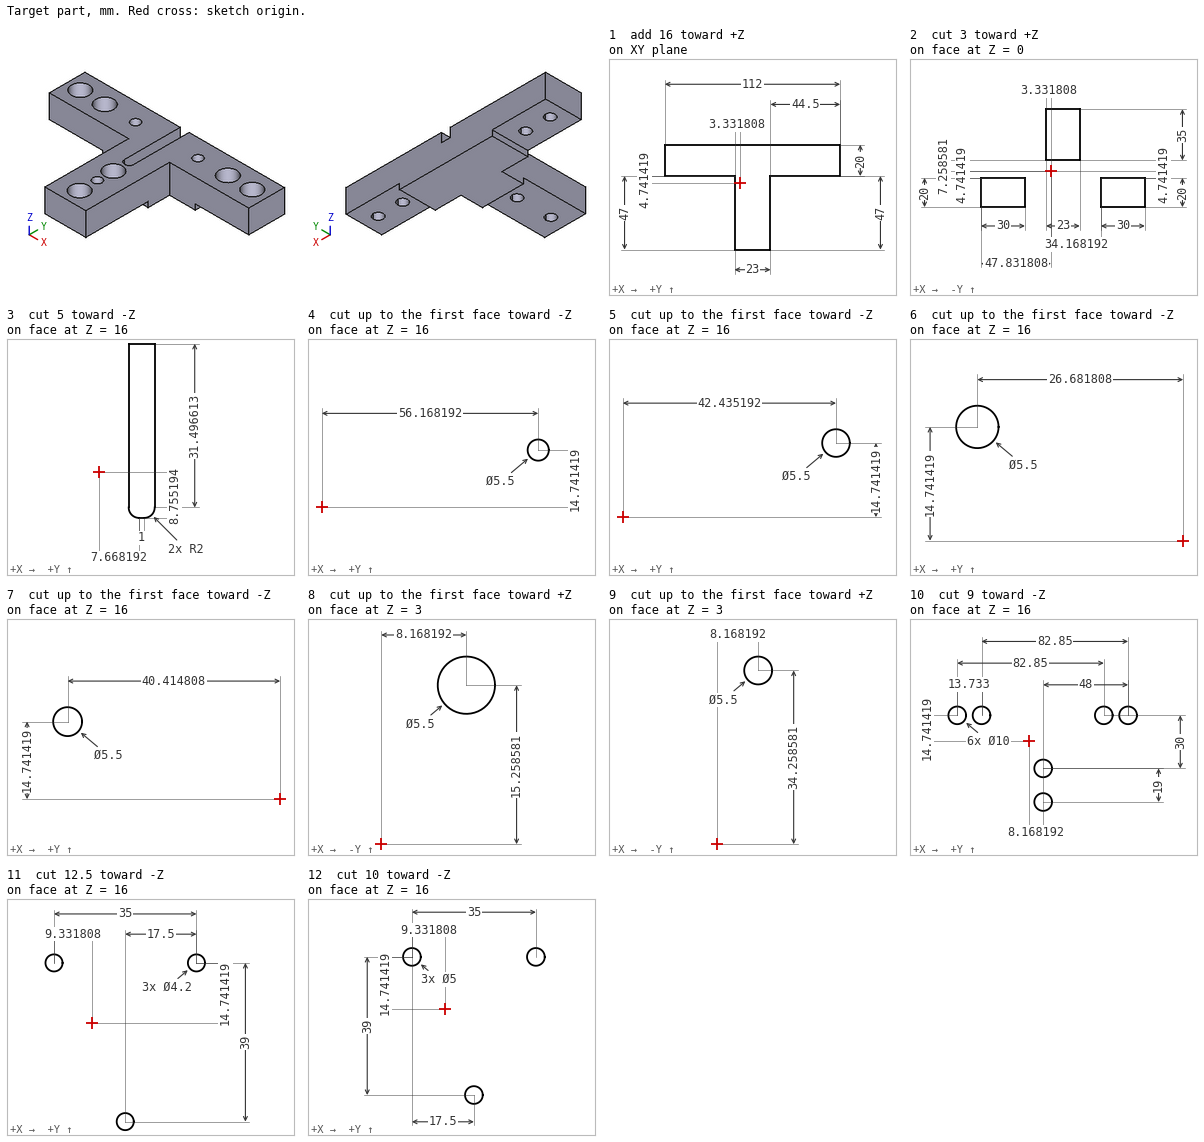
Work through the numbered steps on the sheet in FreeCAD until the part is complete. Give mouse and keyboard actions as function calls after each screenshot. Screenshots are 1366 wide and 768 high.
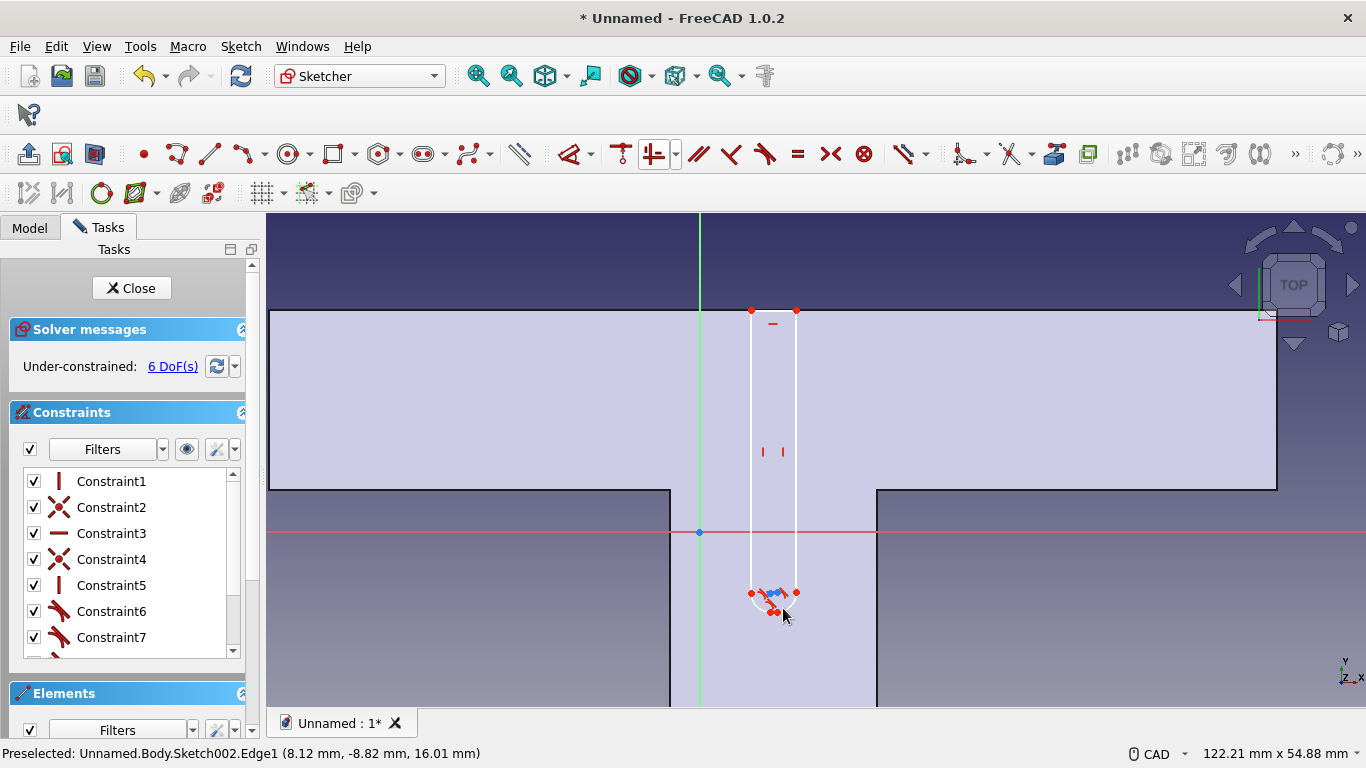
scroll(786, 610, up, 3)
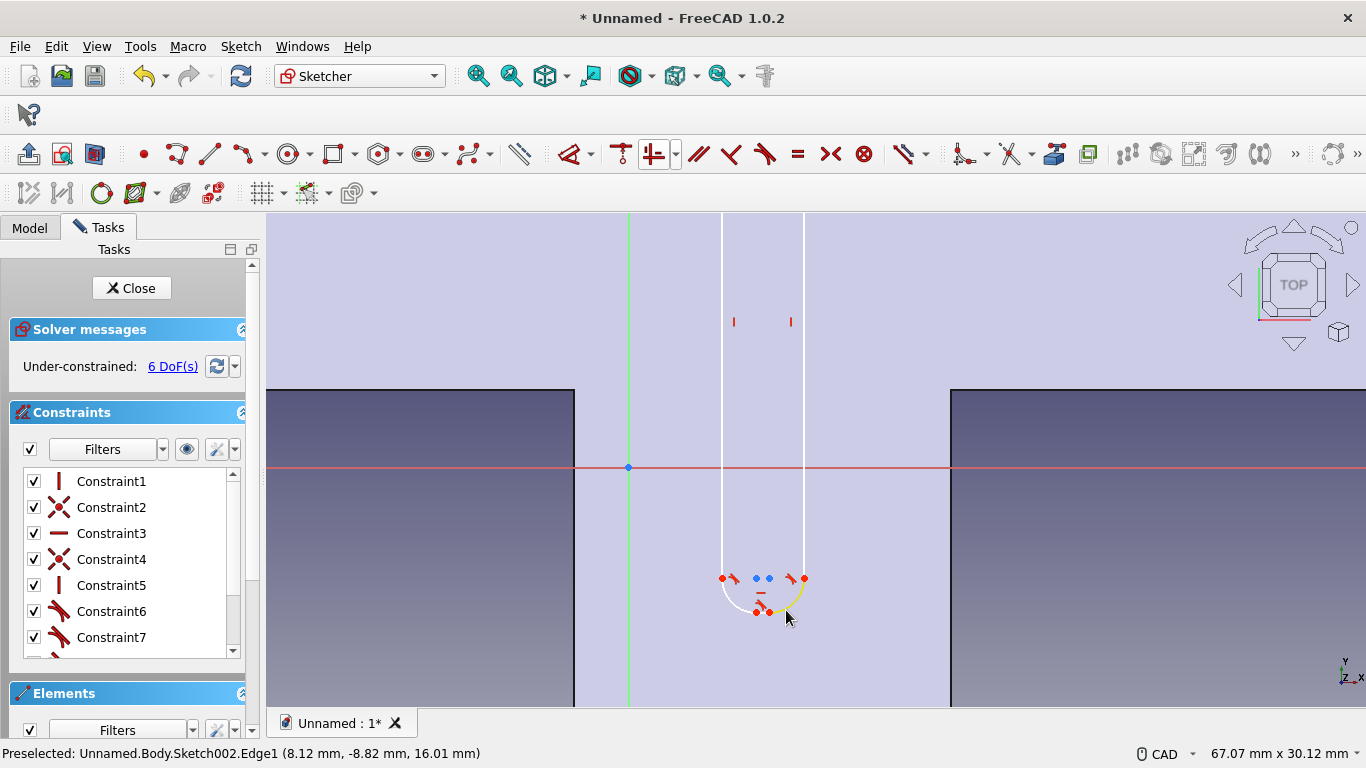
click(785, 609)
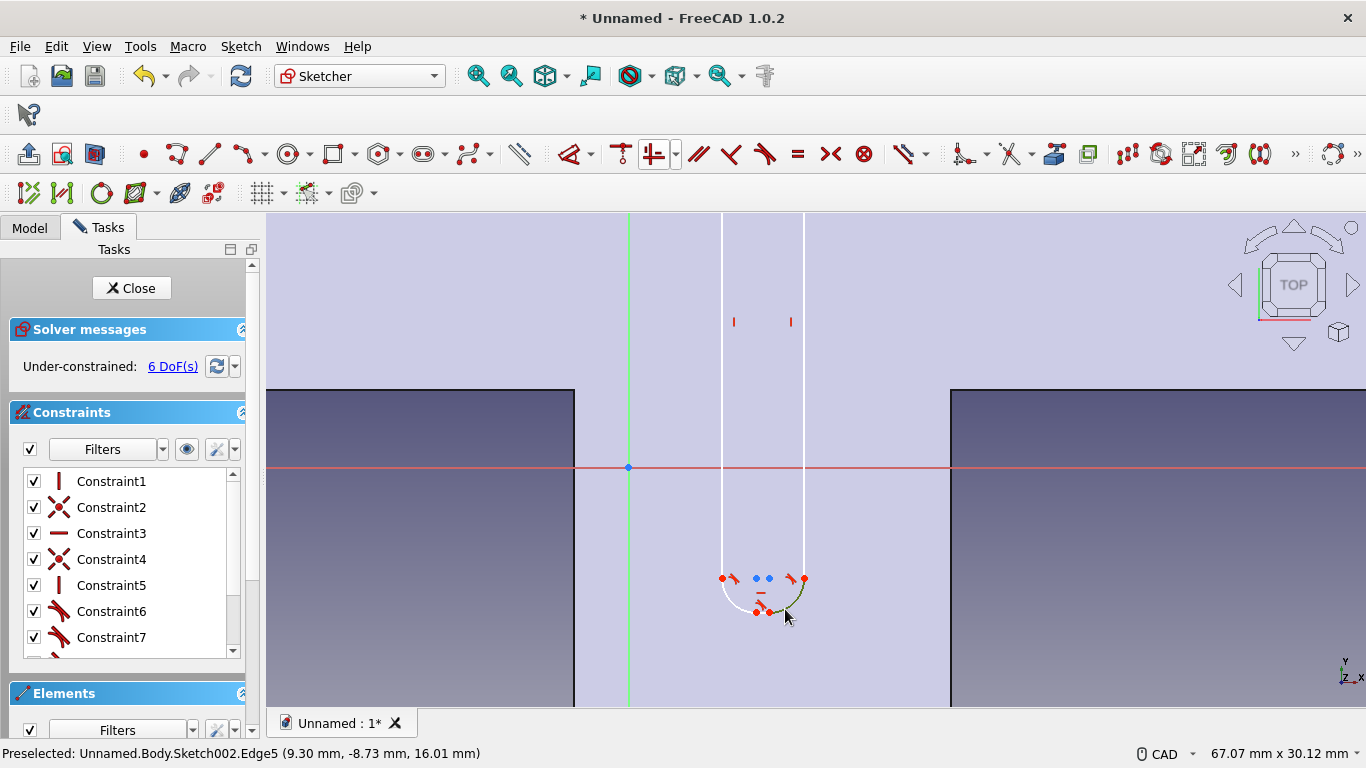
click(726, 594)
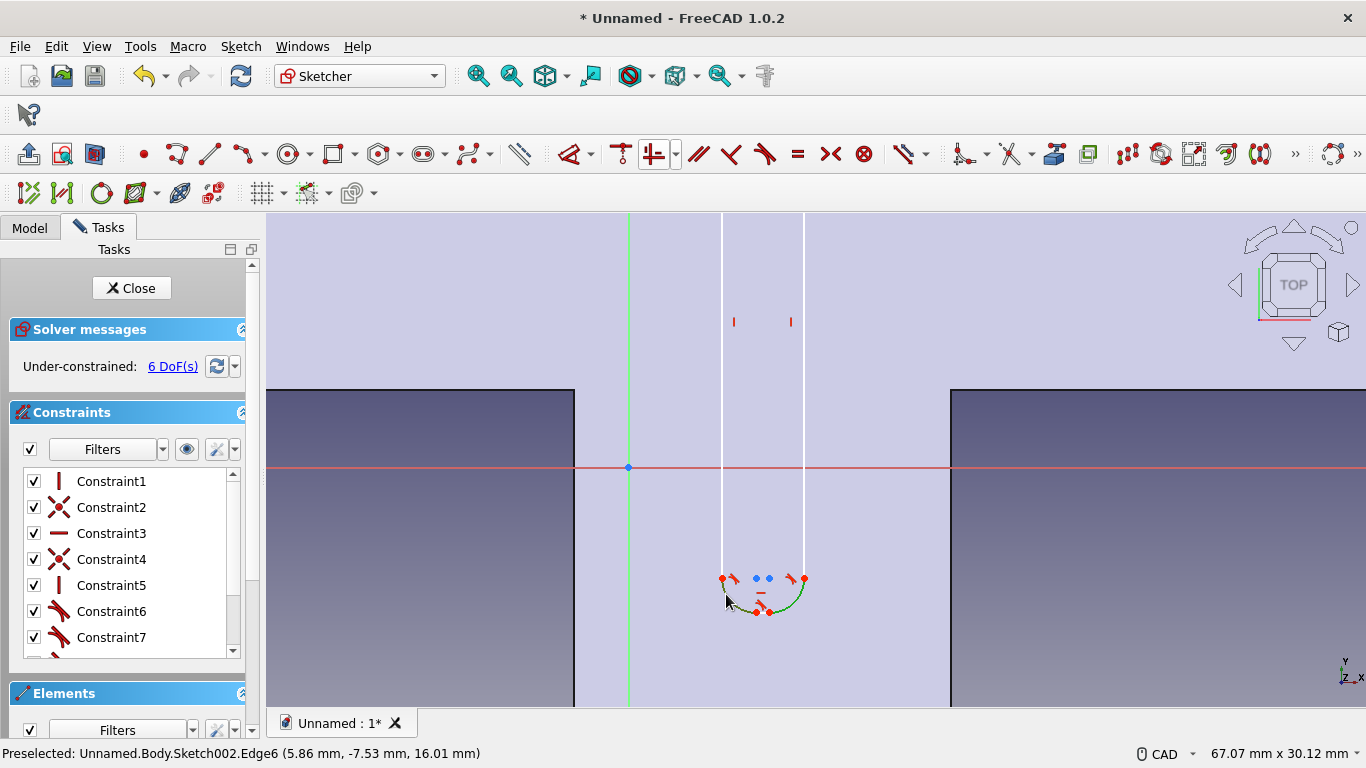
click(798, 154)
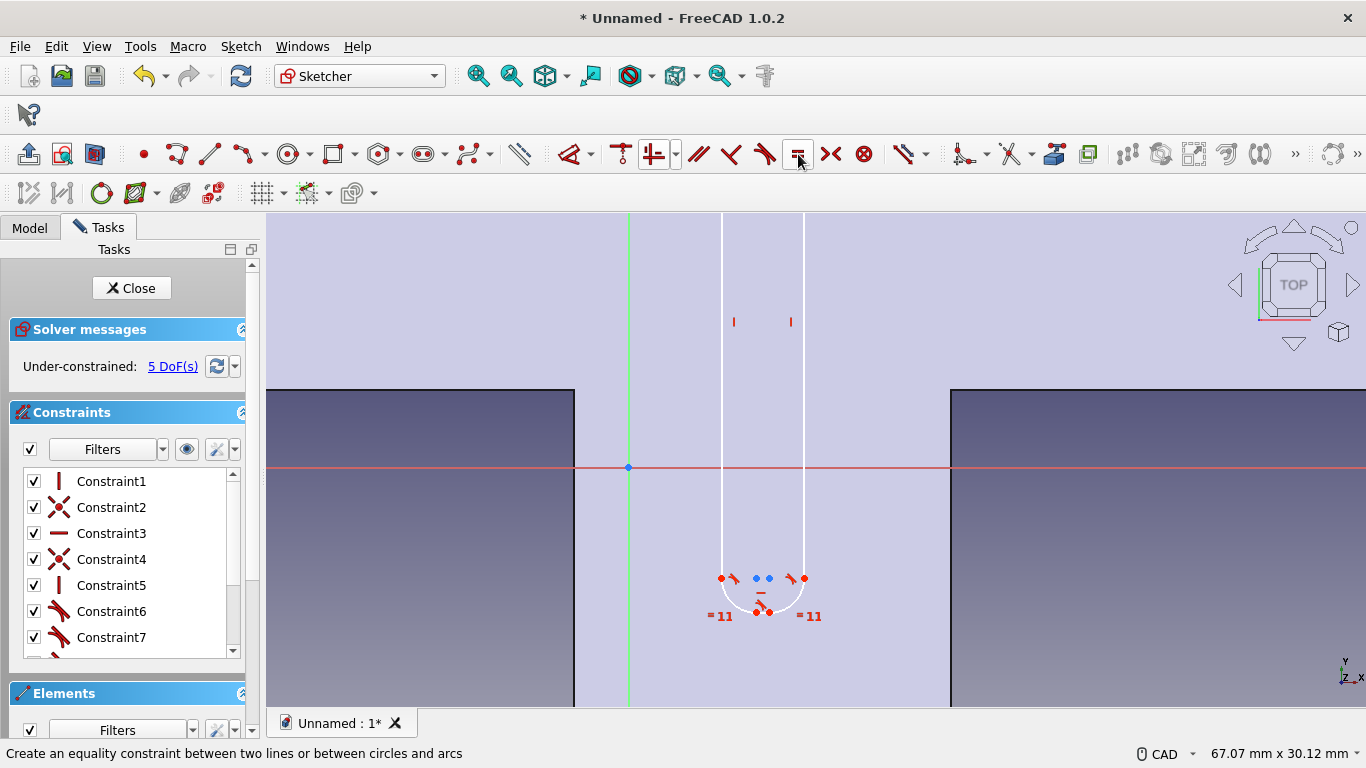
click(568, 154)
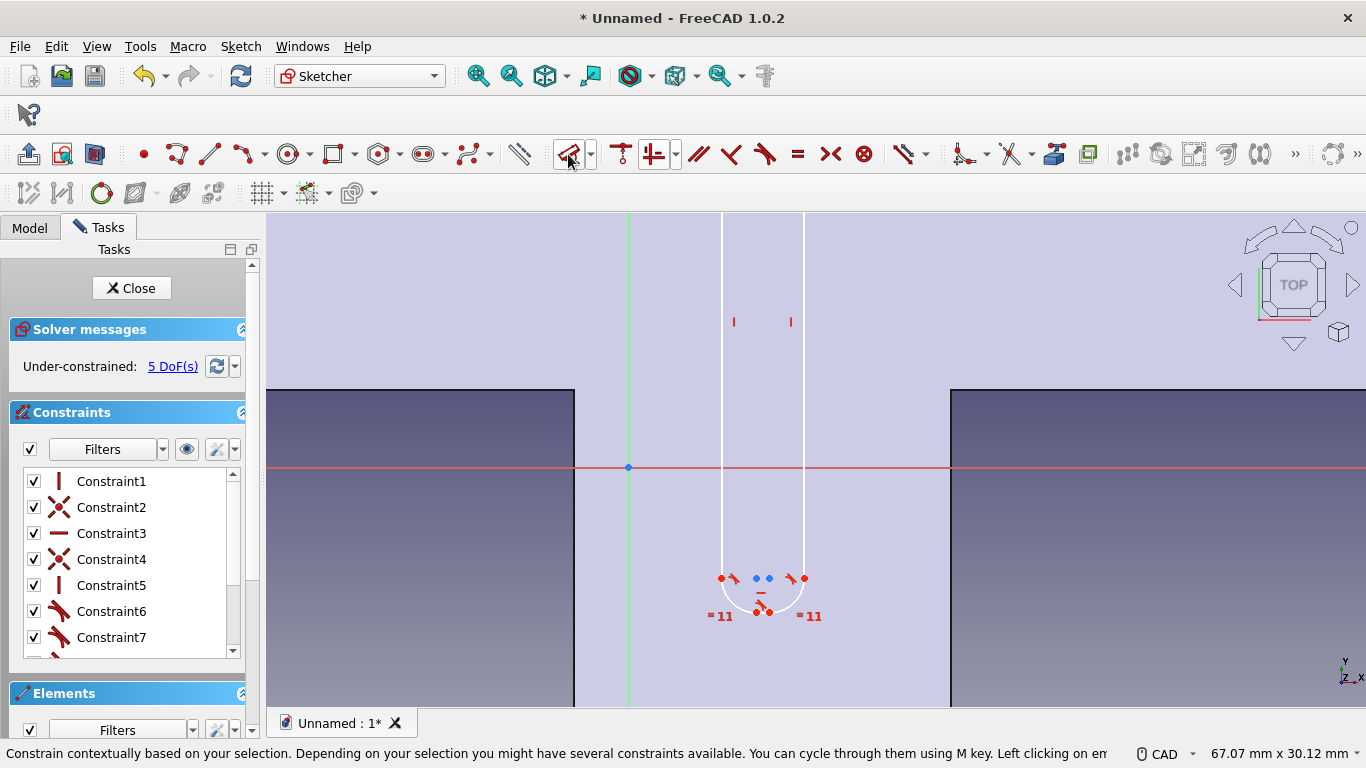
click(785, 609)
click(799, 638)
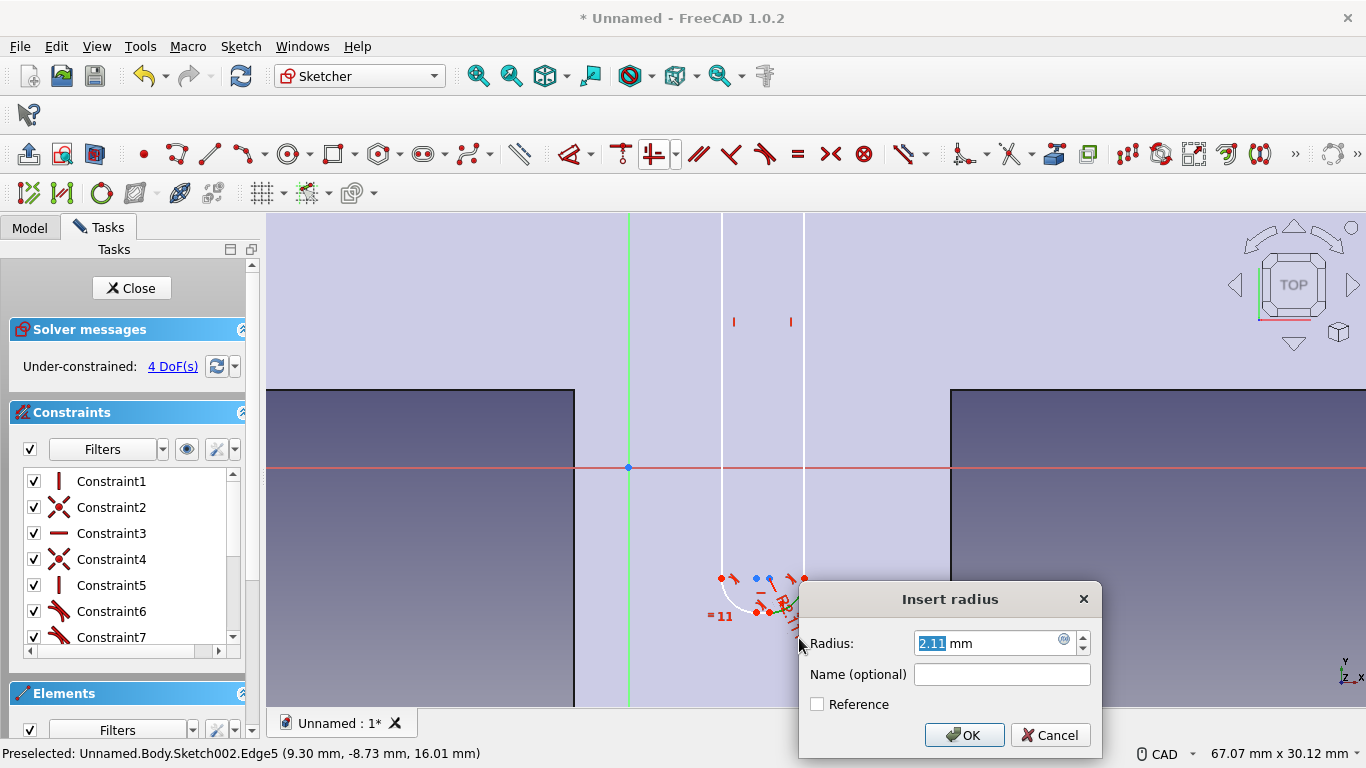
text(2)
key(Return)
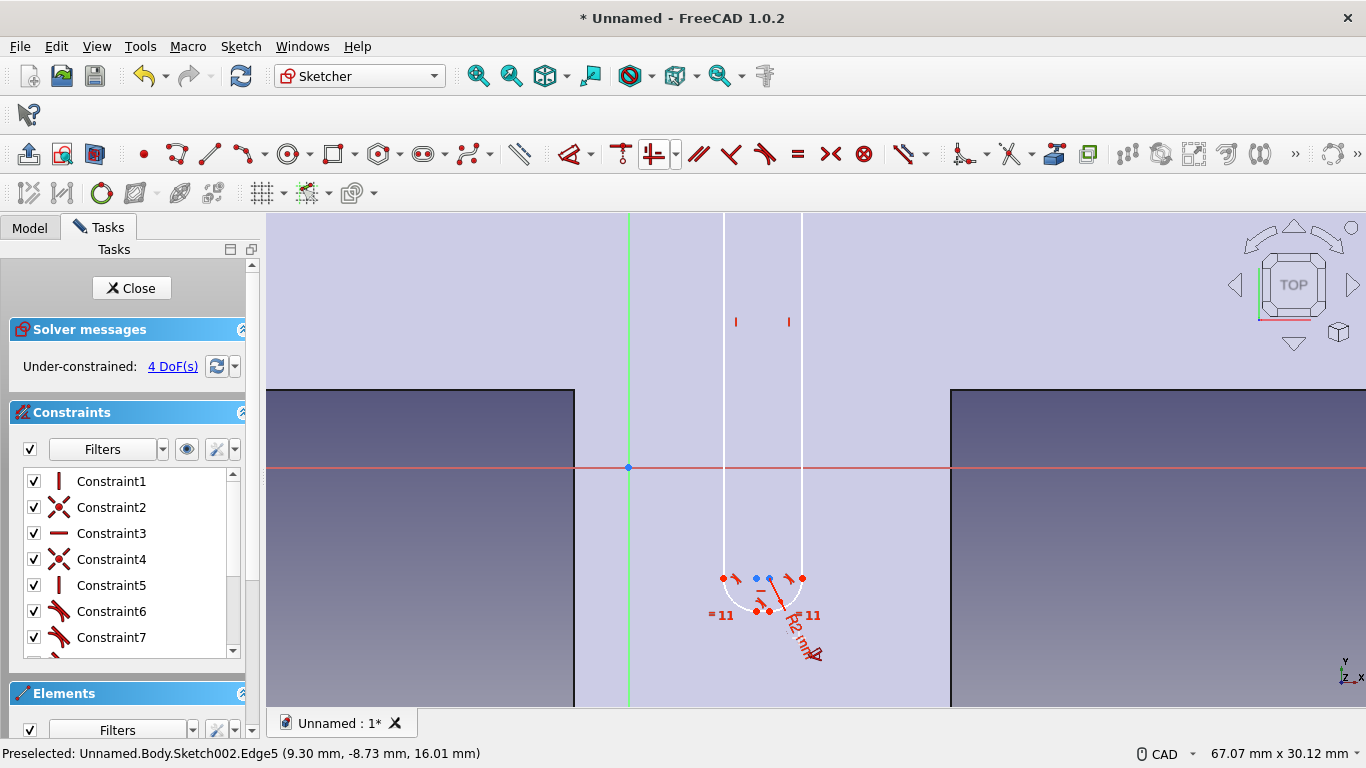
scroll(763, 611, up, 5)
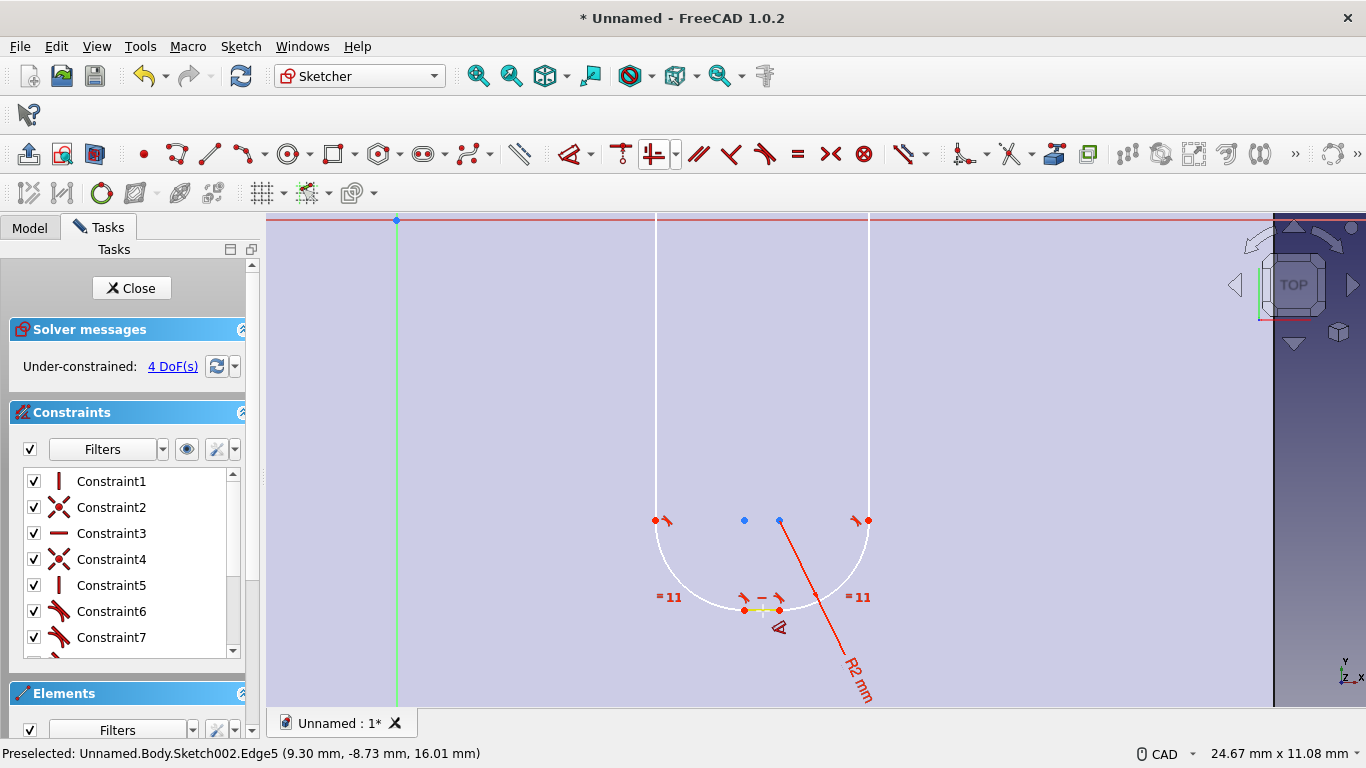
click(762, 610)
click(762, 644)